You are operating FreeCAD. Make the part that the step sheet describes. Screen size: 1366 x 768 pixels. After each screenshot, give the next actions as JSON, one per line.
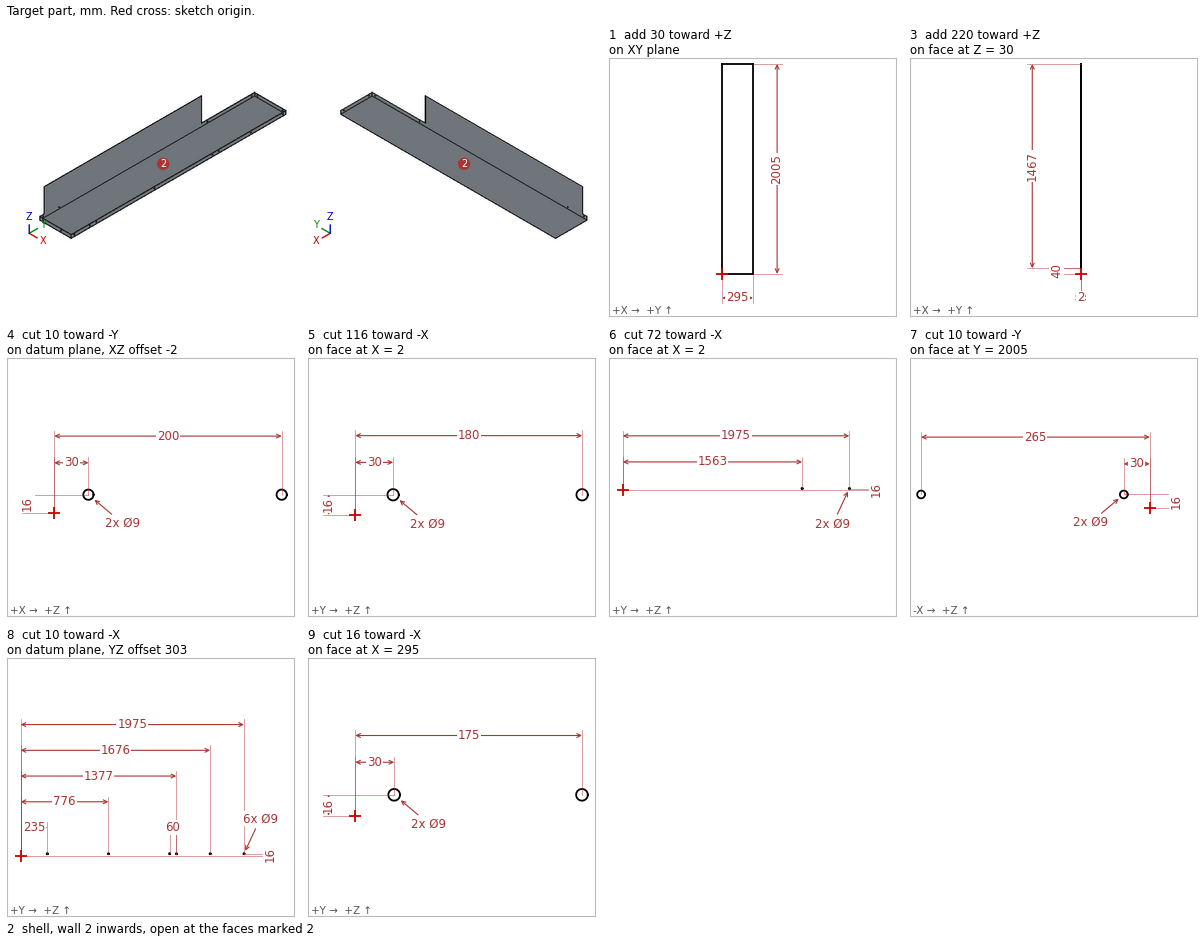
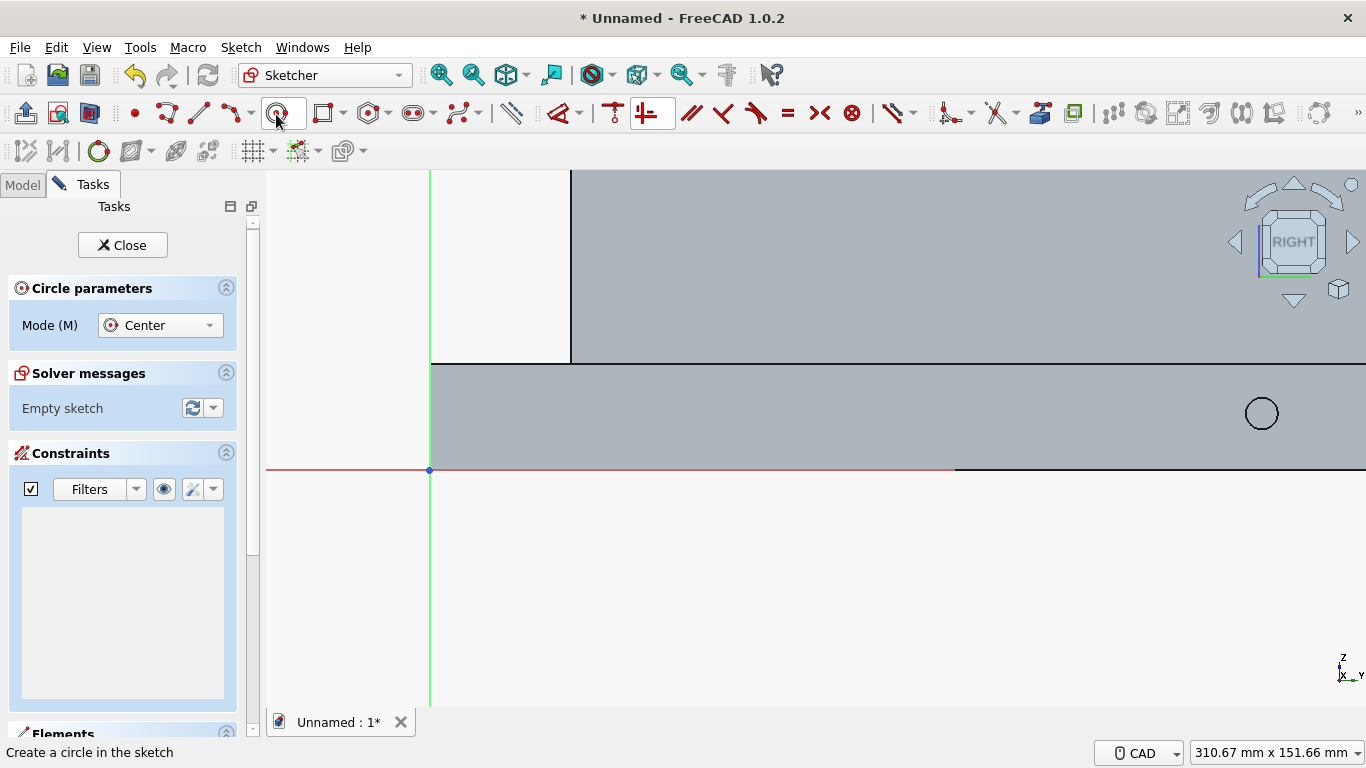
{"action": "scroll", "coordinate": [536, 414], "scroll_direction": "up", "scroll_amount": 2}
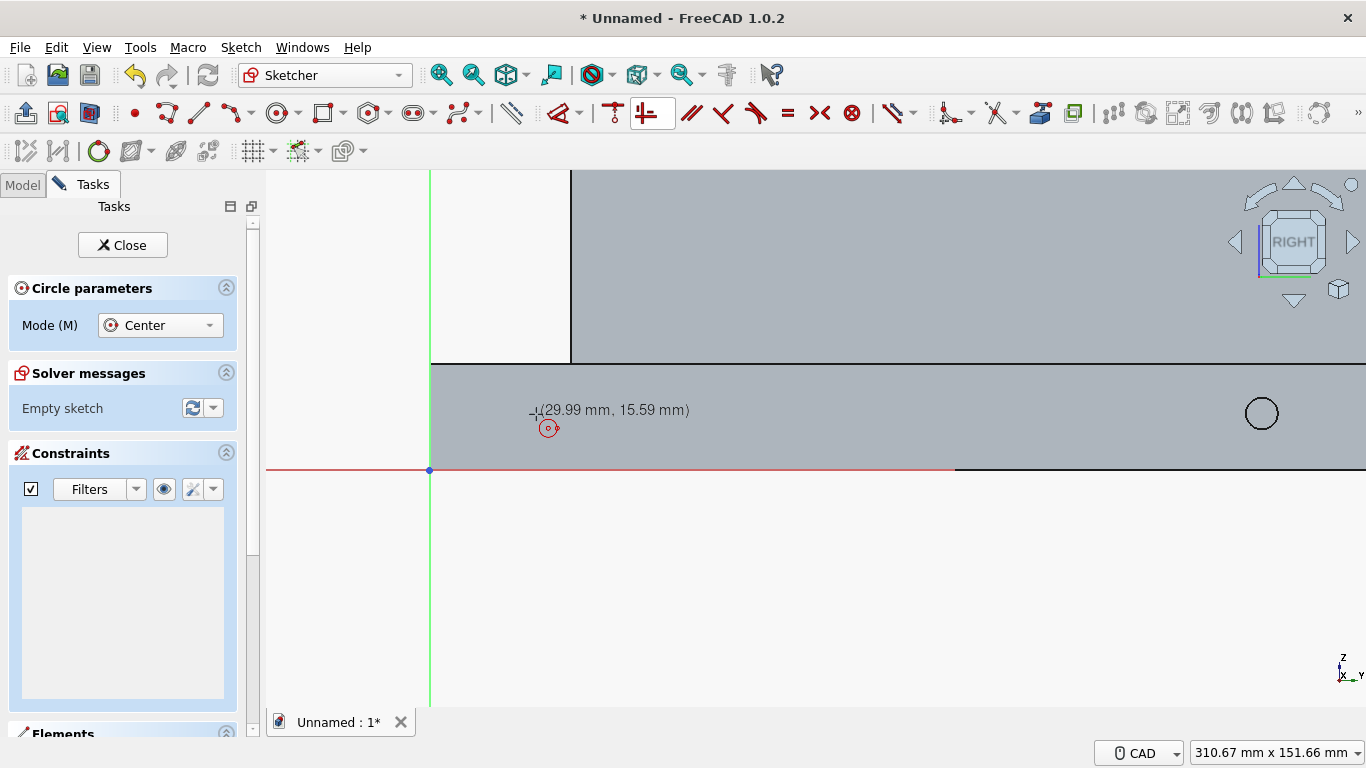
{"action": "left_click", "coordinate": [536, 413]}
{"action": "left_click", "coordinate": [553, 396]}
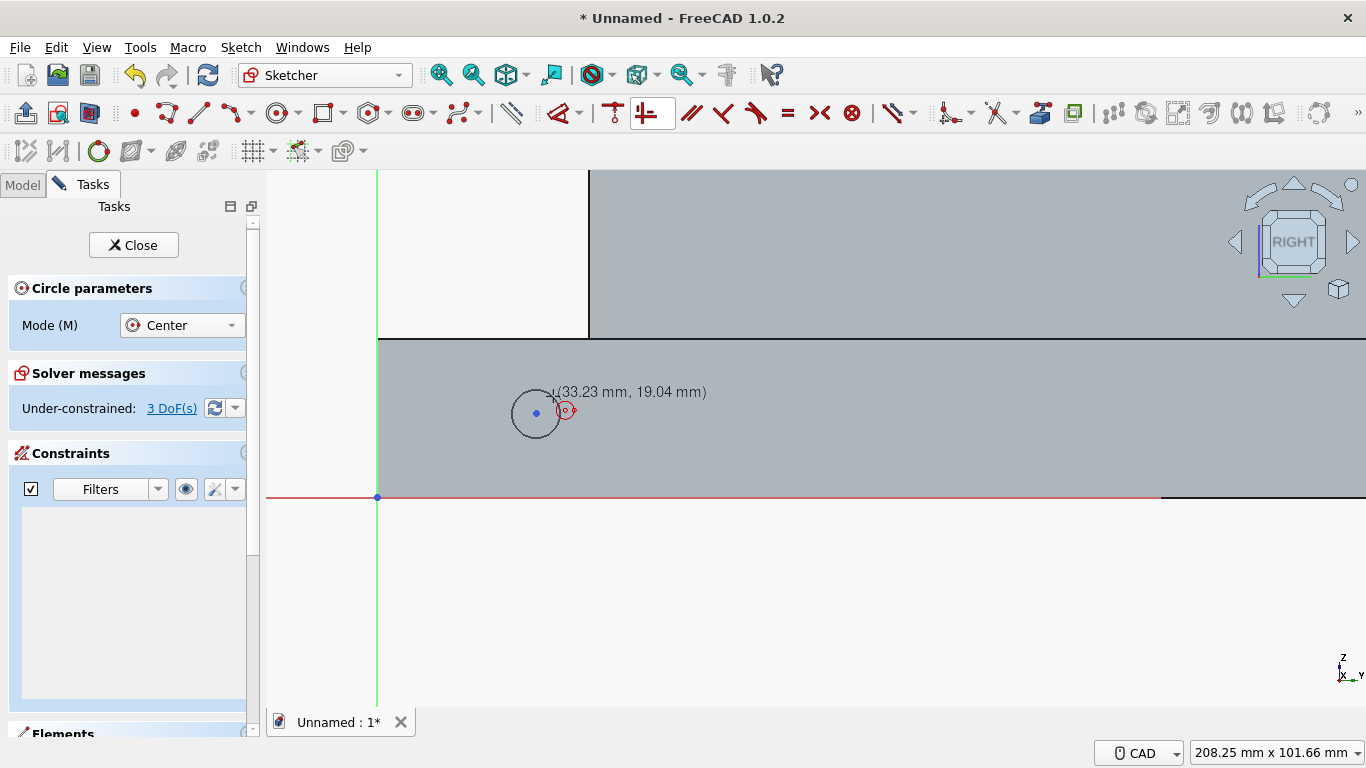
{"action": "scroll", "coordinate": [536, 428], "scroll_direction": "down", "scroll_amount": 2}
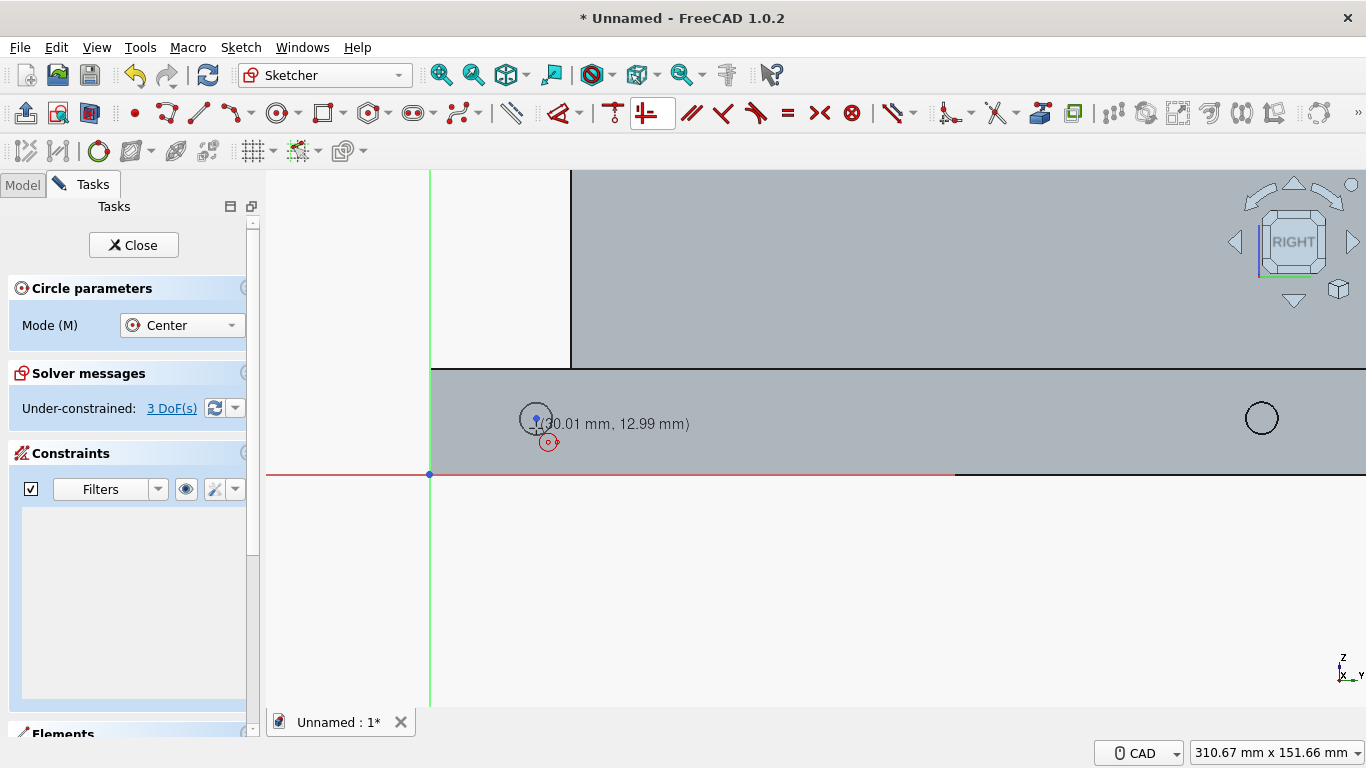
{"action": "scroll", "coordinate": [1049, 418], "scroll_direction": "up", "scroll_amount": 2}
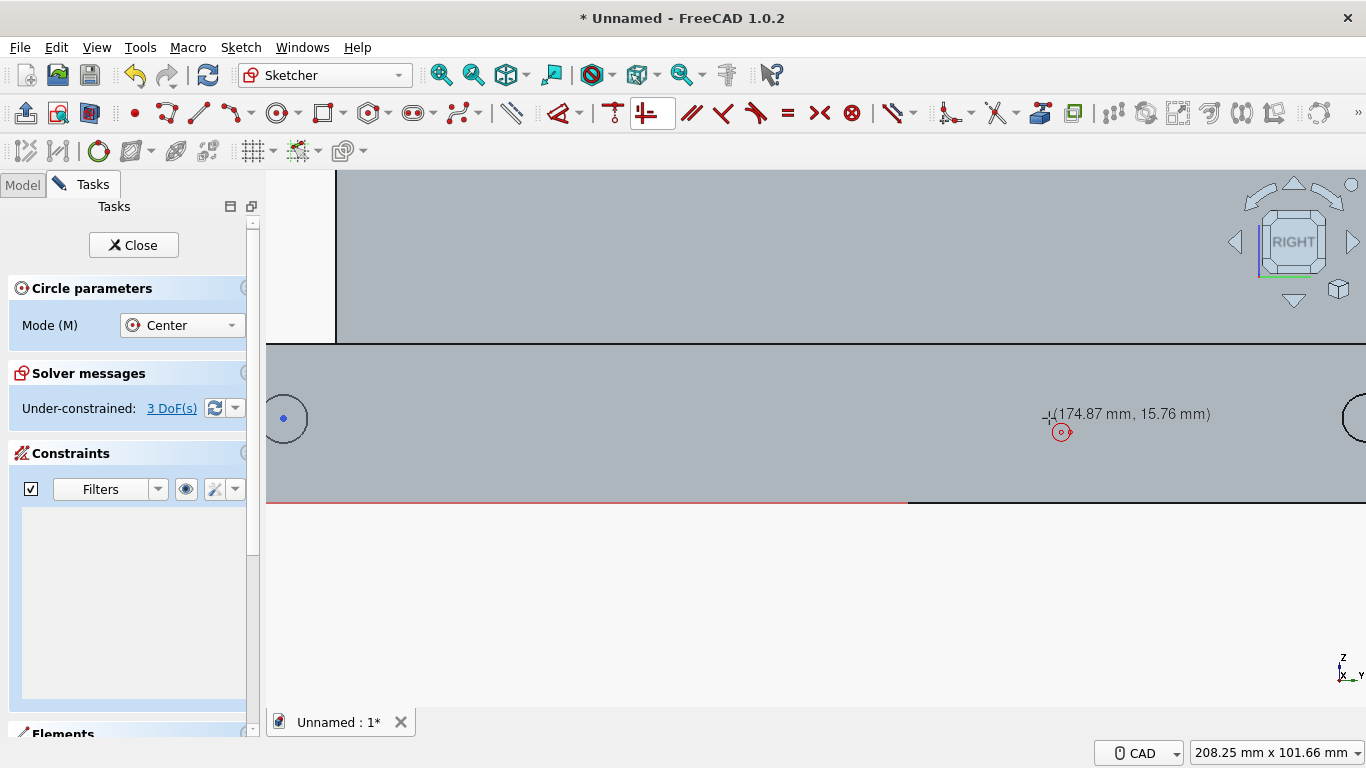
{"action": "left_click", "coordinate": [1049, 418]}
{"action": "left_click", "coordinate": [1066, 401]}
{"action": "key", "text": "Escape"}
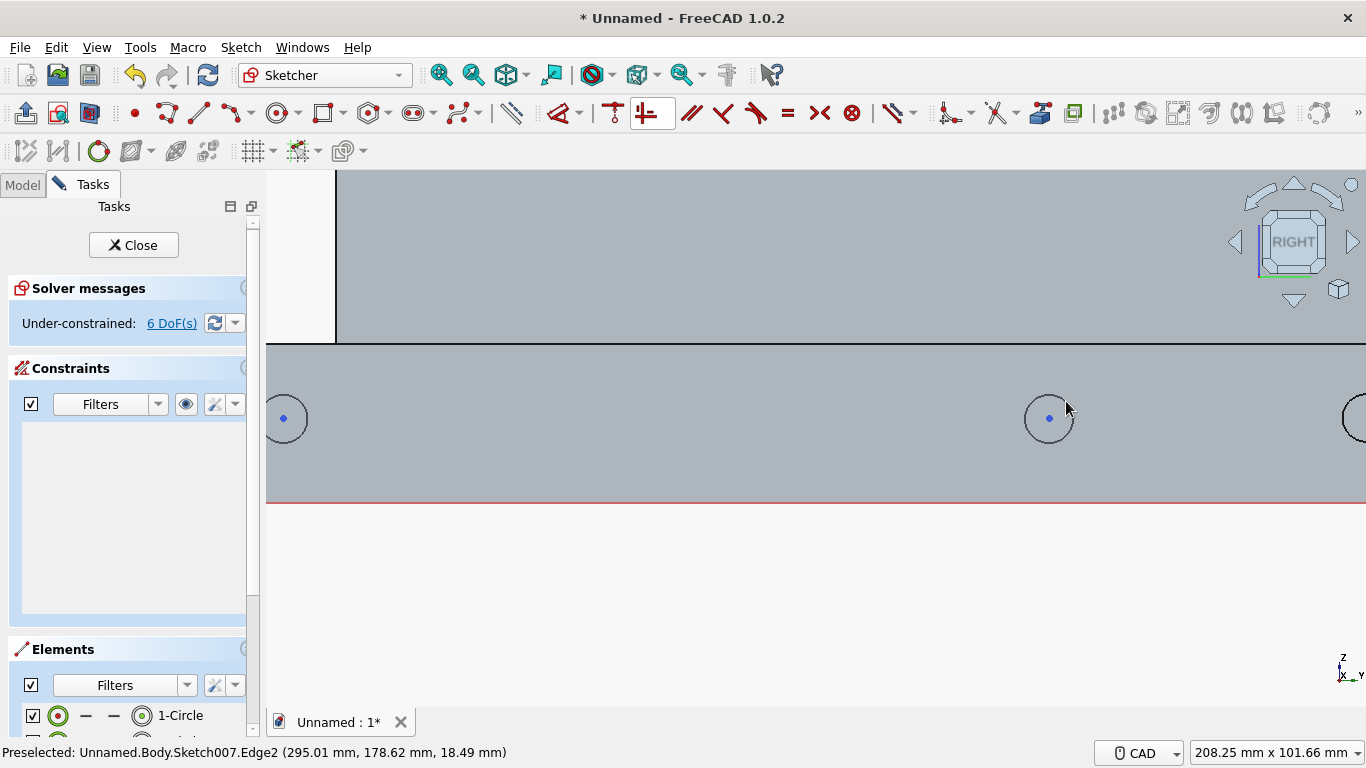
{"action": "left_click", "coordinate": [300, 402]}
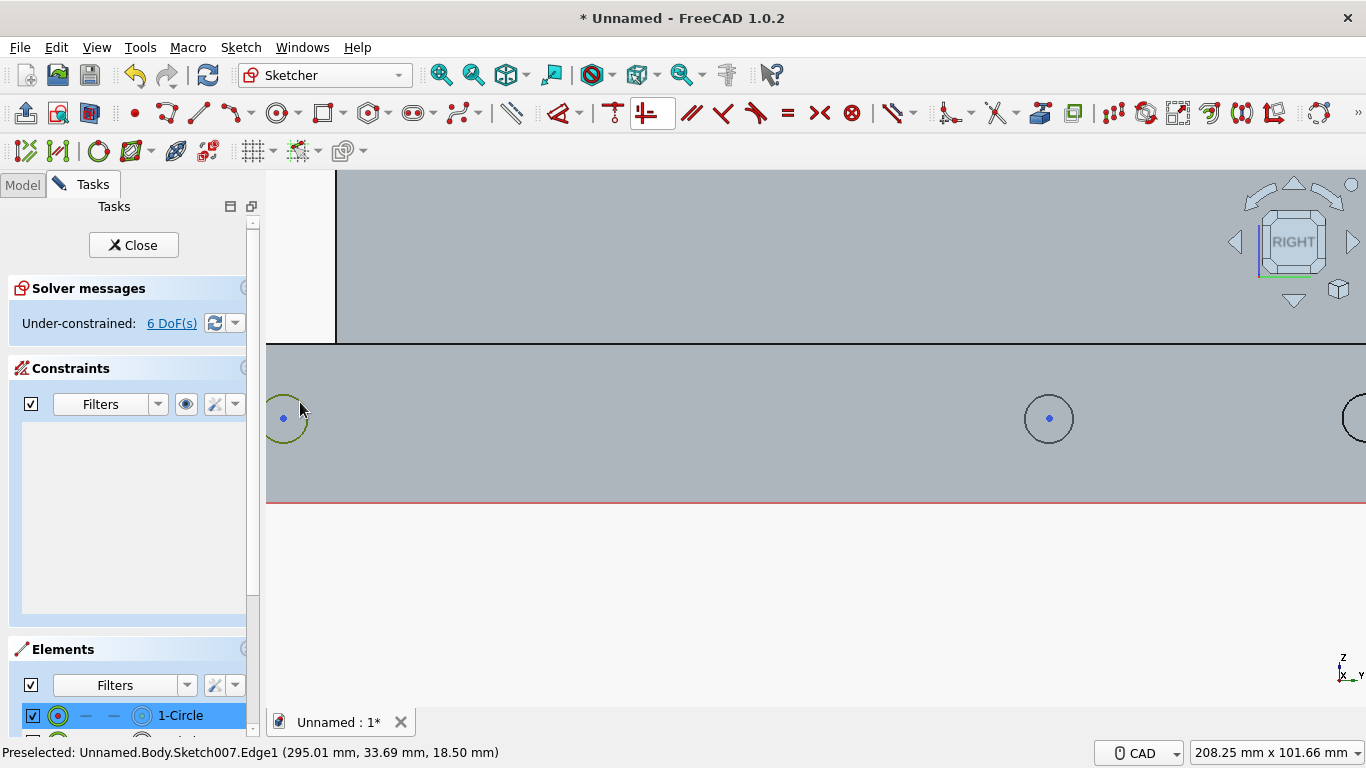
{"action": "left_click", "coordinate": [1066, 402]}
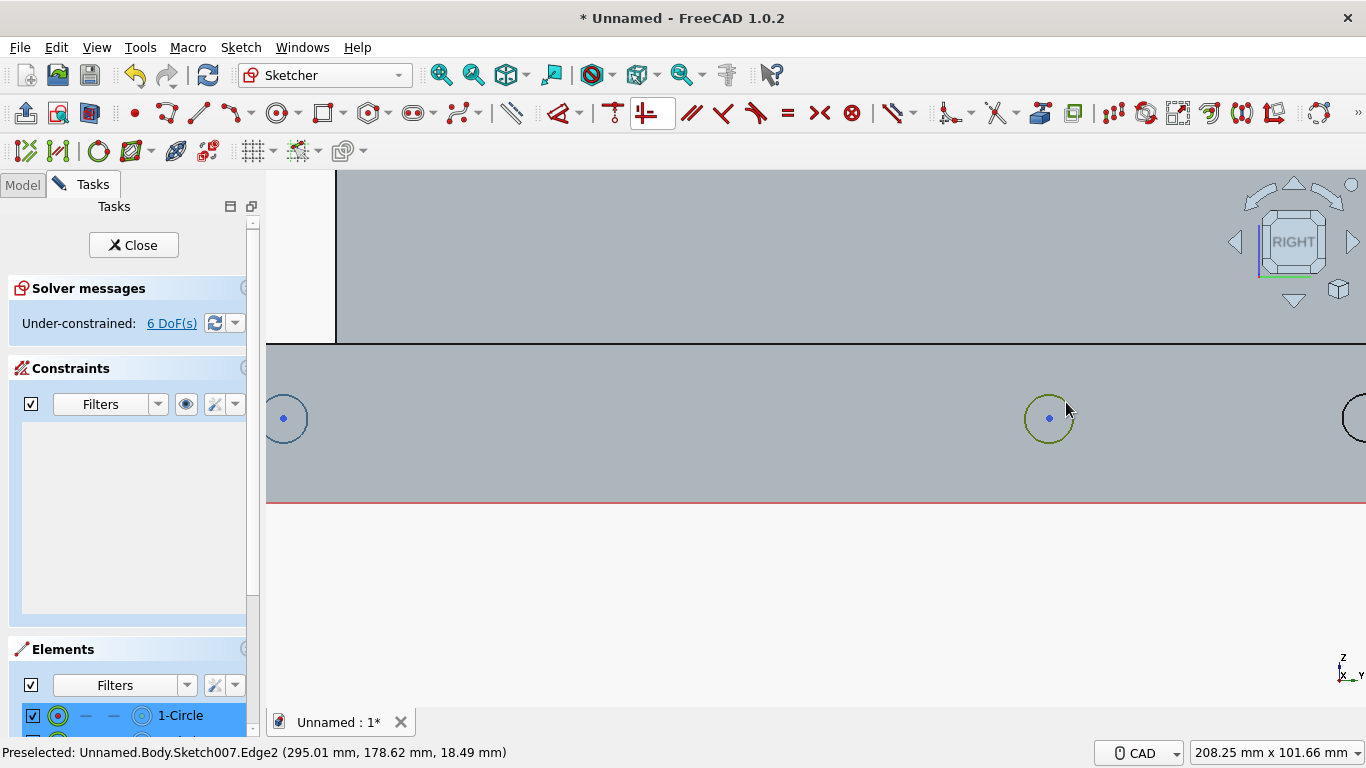
{"action": "left_click", "coordinate": [788, 114]}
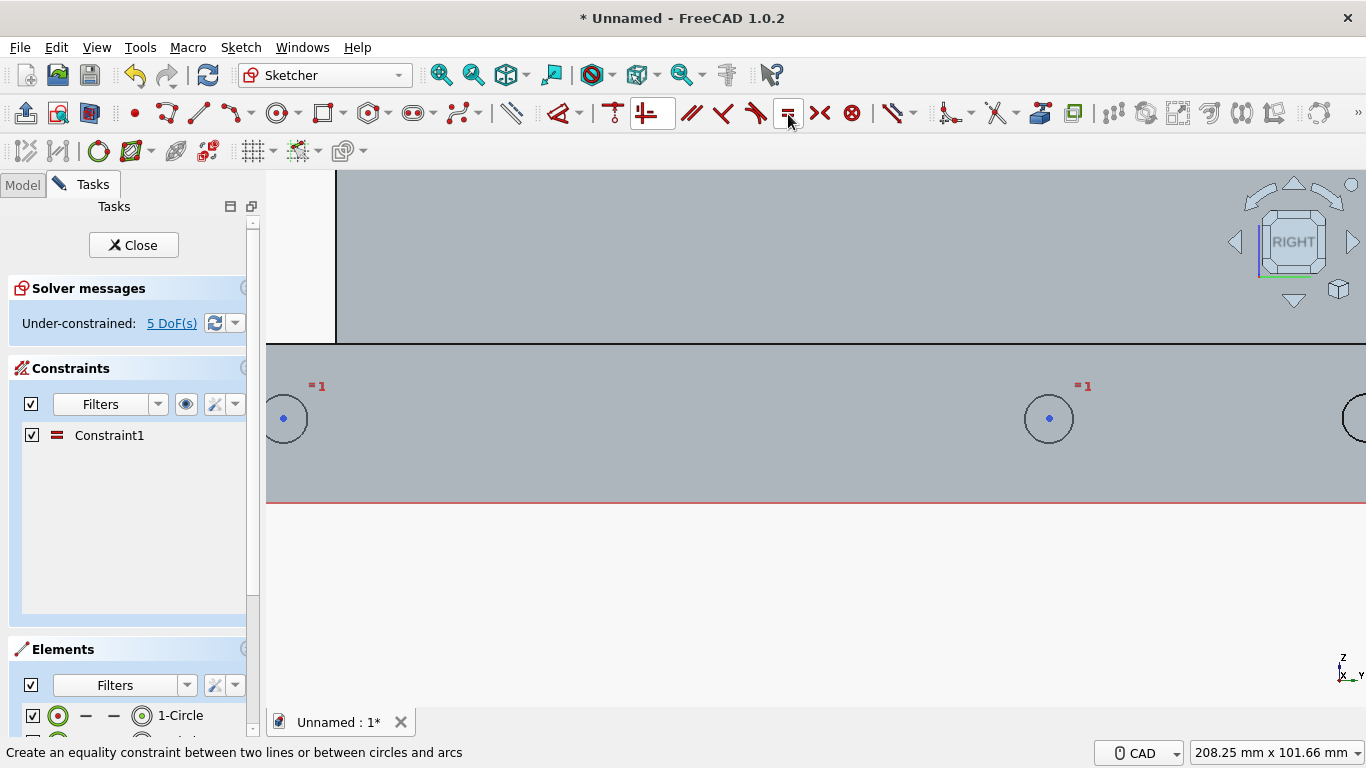
{"action": "scroll", "coordinate": [1049, 418], "scroll_direction": "down", "scroll_amount": 2}